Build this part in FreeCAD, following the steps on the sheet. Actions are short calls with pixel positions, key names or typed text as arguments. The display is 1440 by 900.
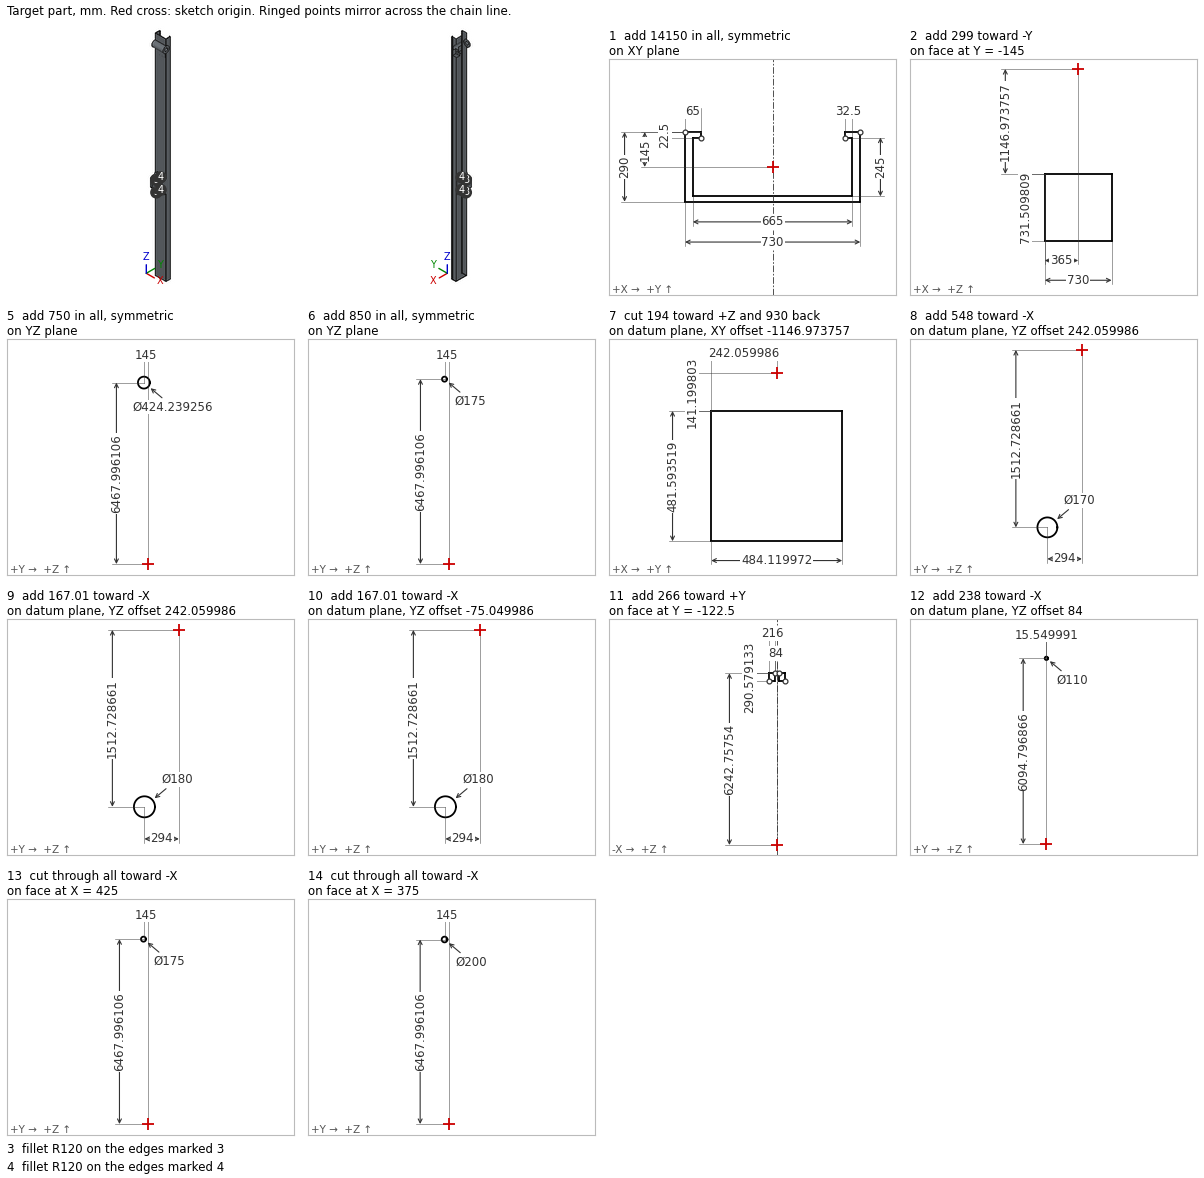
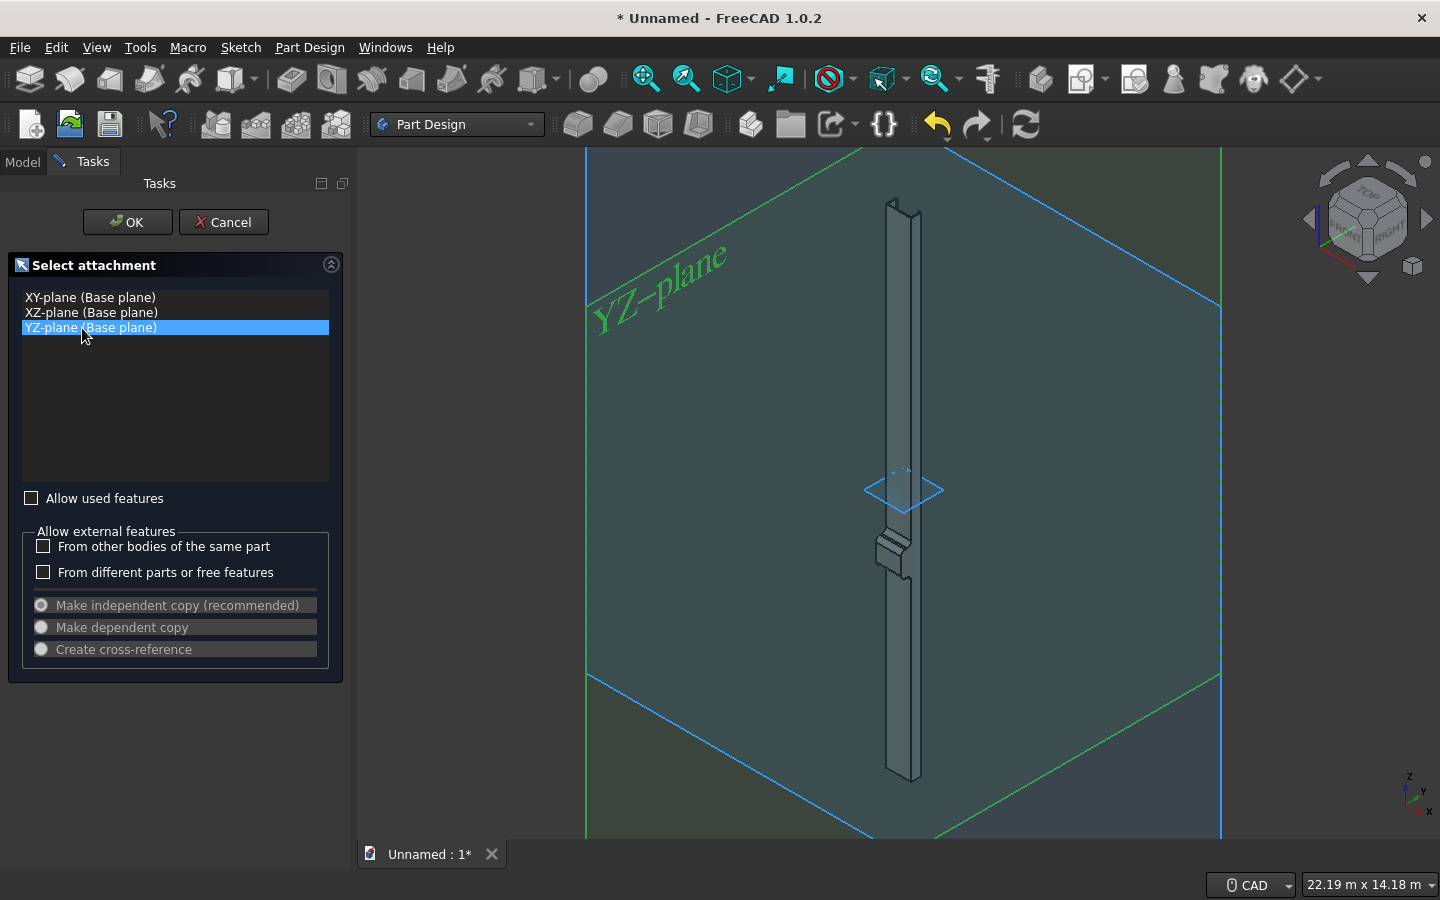
click(128, 222)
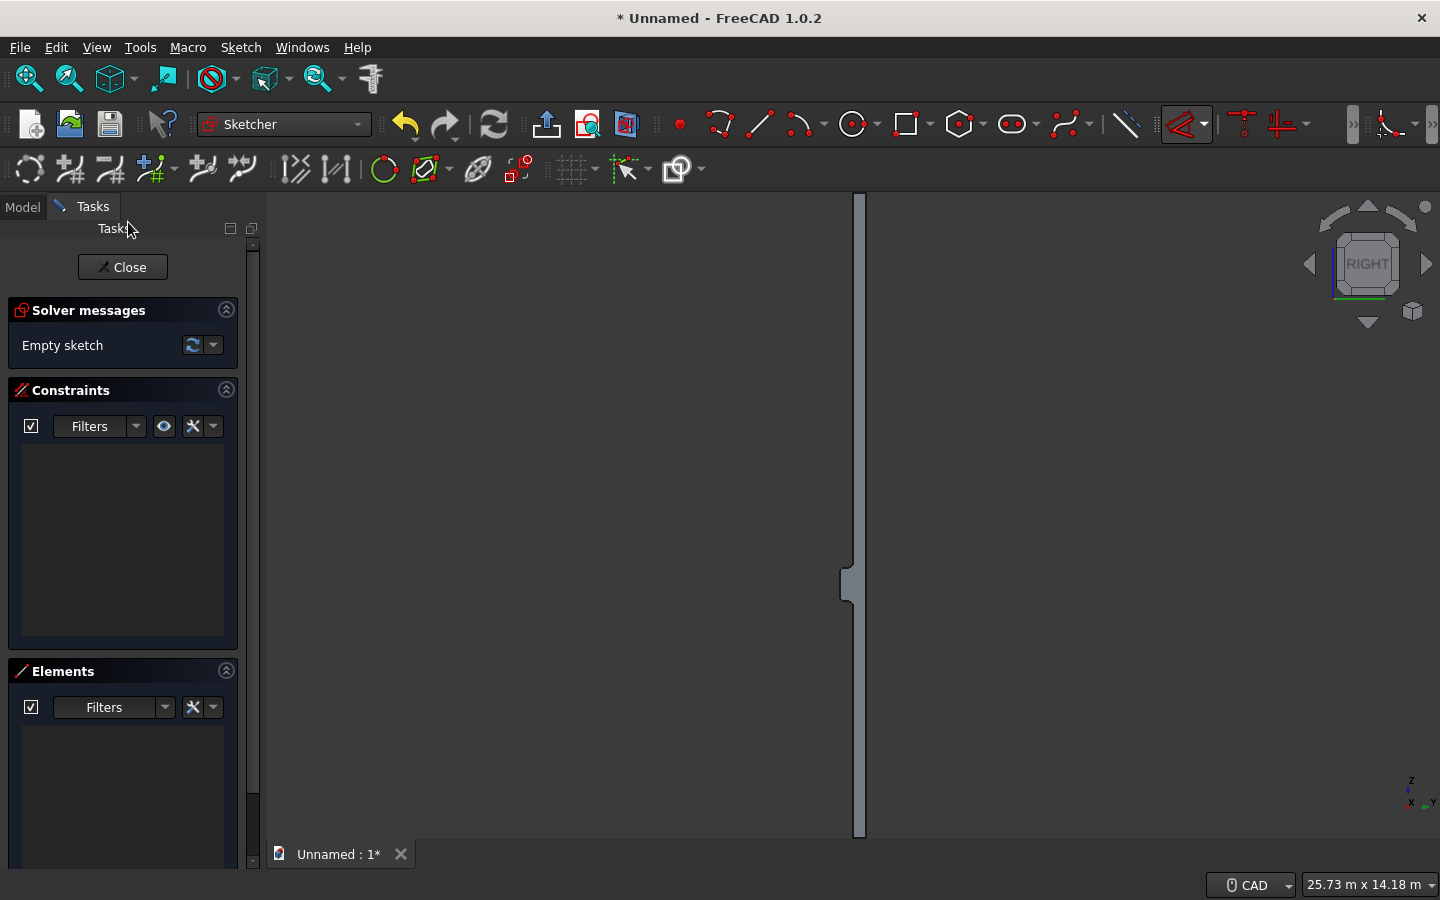
key(q)
key(s)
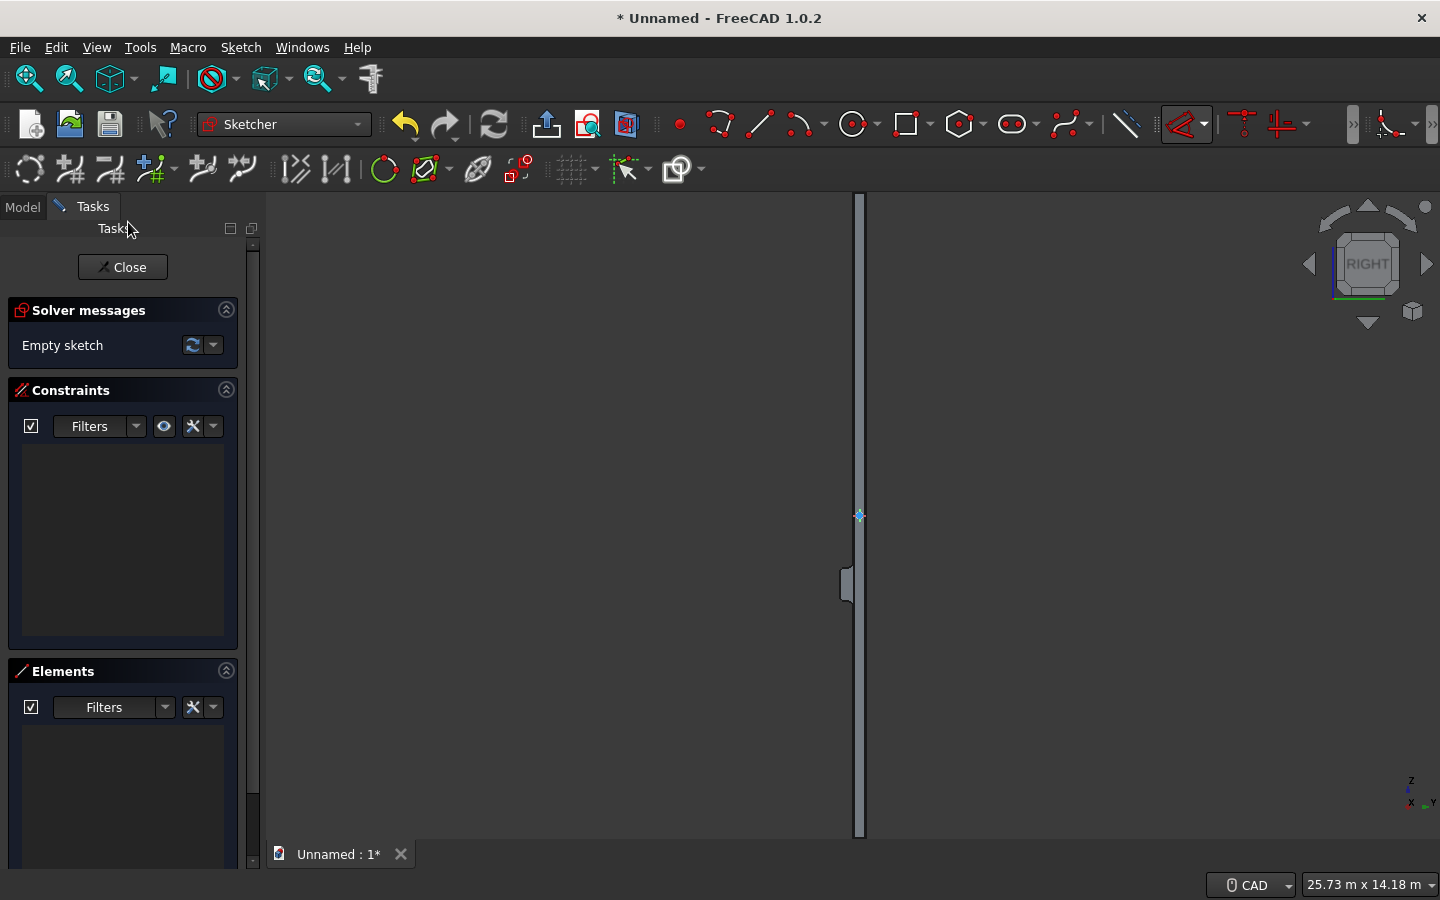
scroll(784, 516, down, 5)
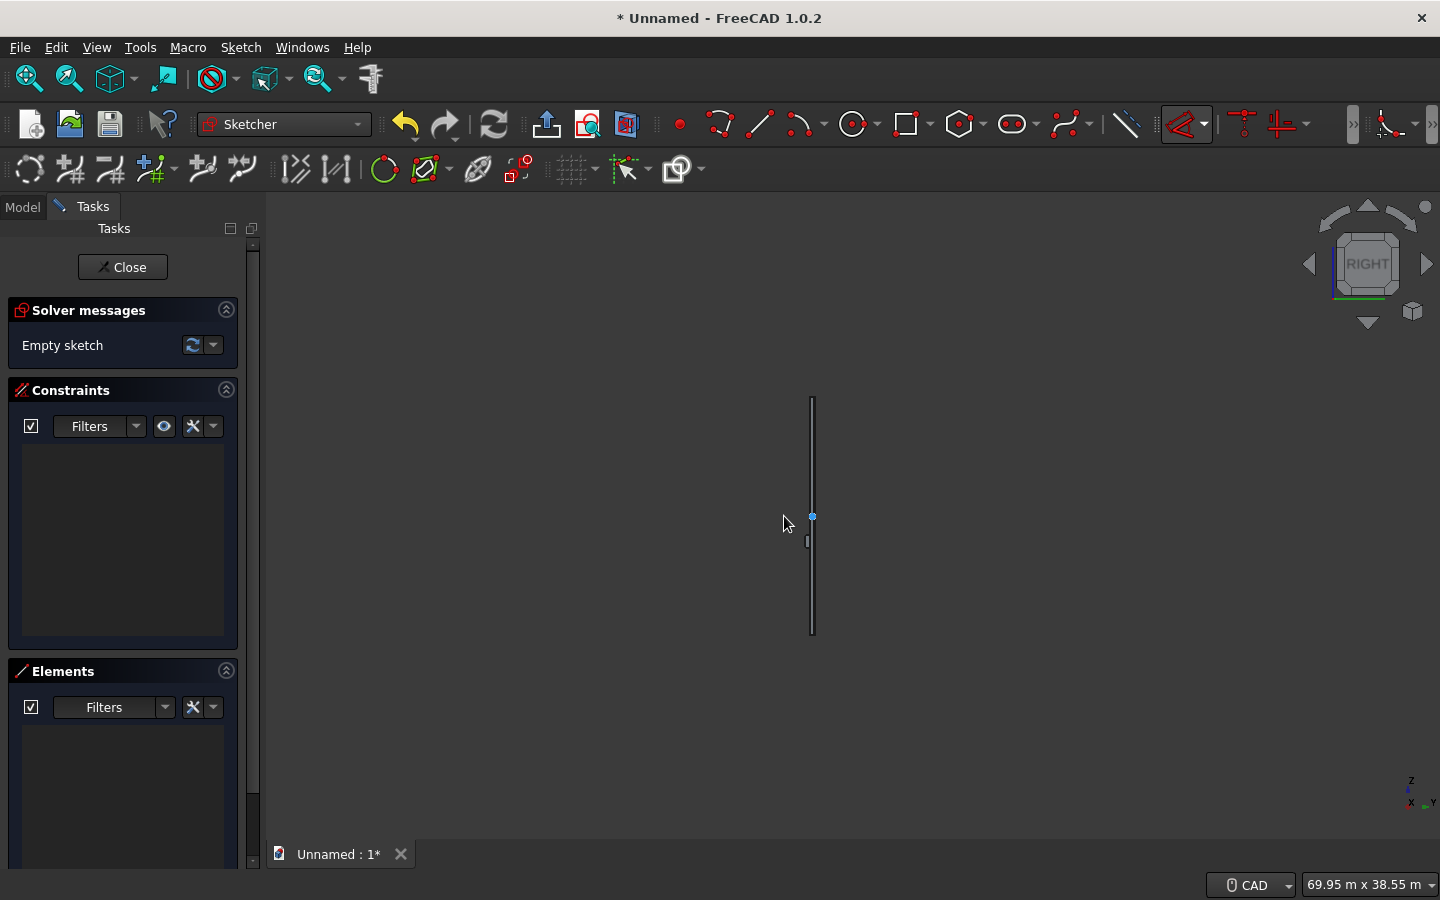
scroll(811, 402, up, 15)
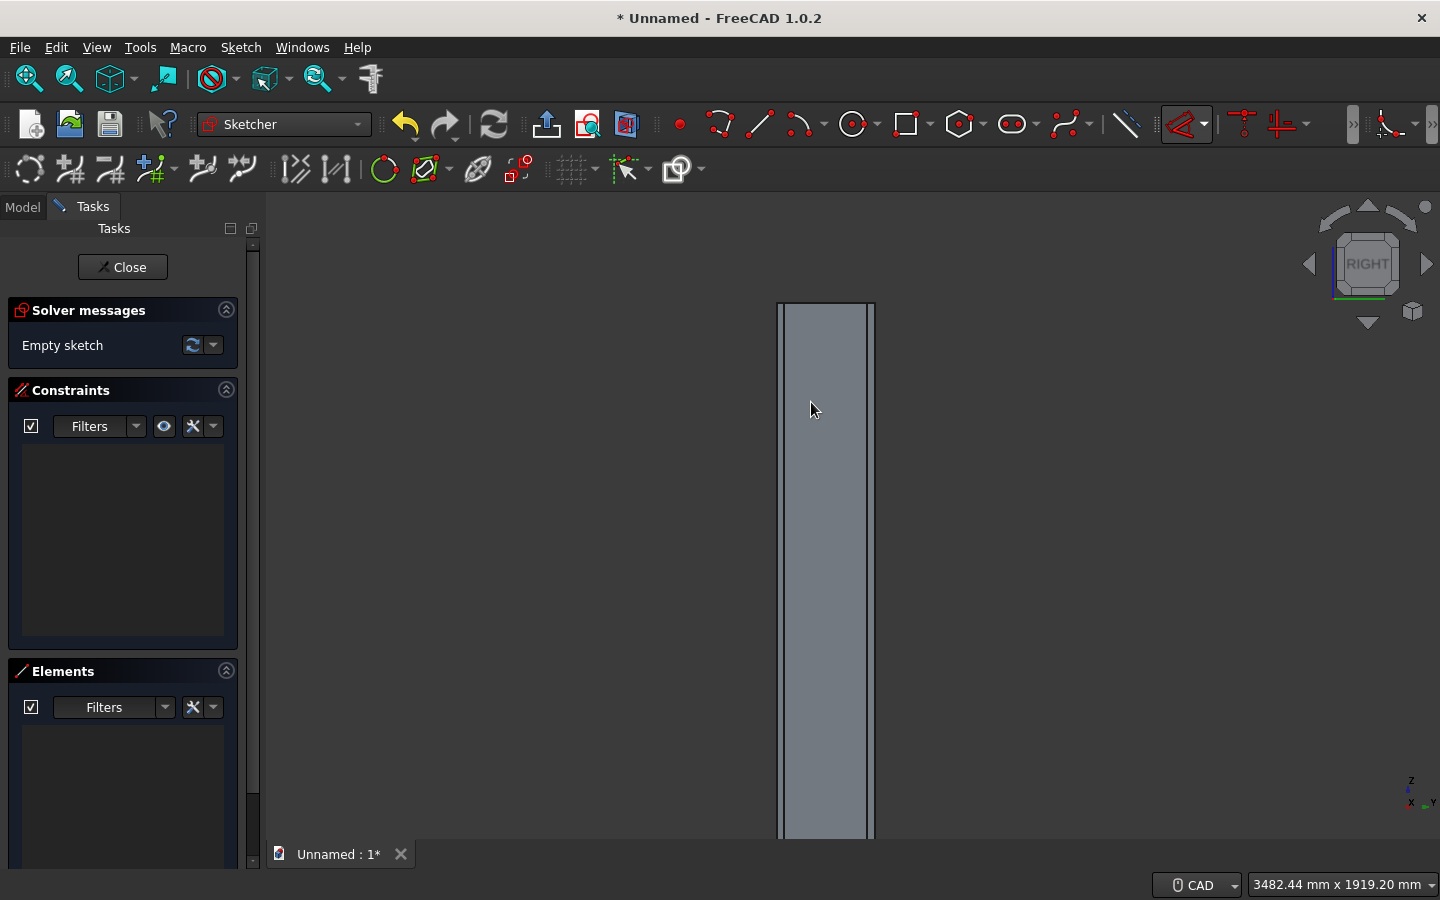
scroll(772, 503, up, 5)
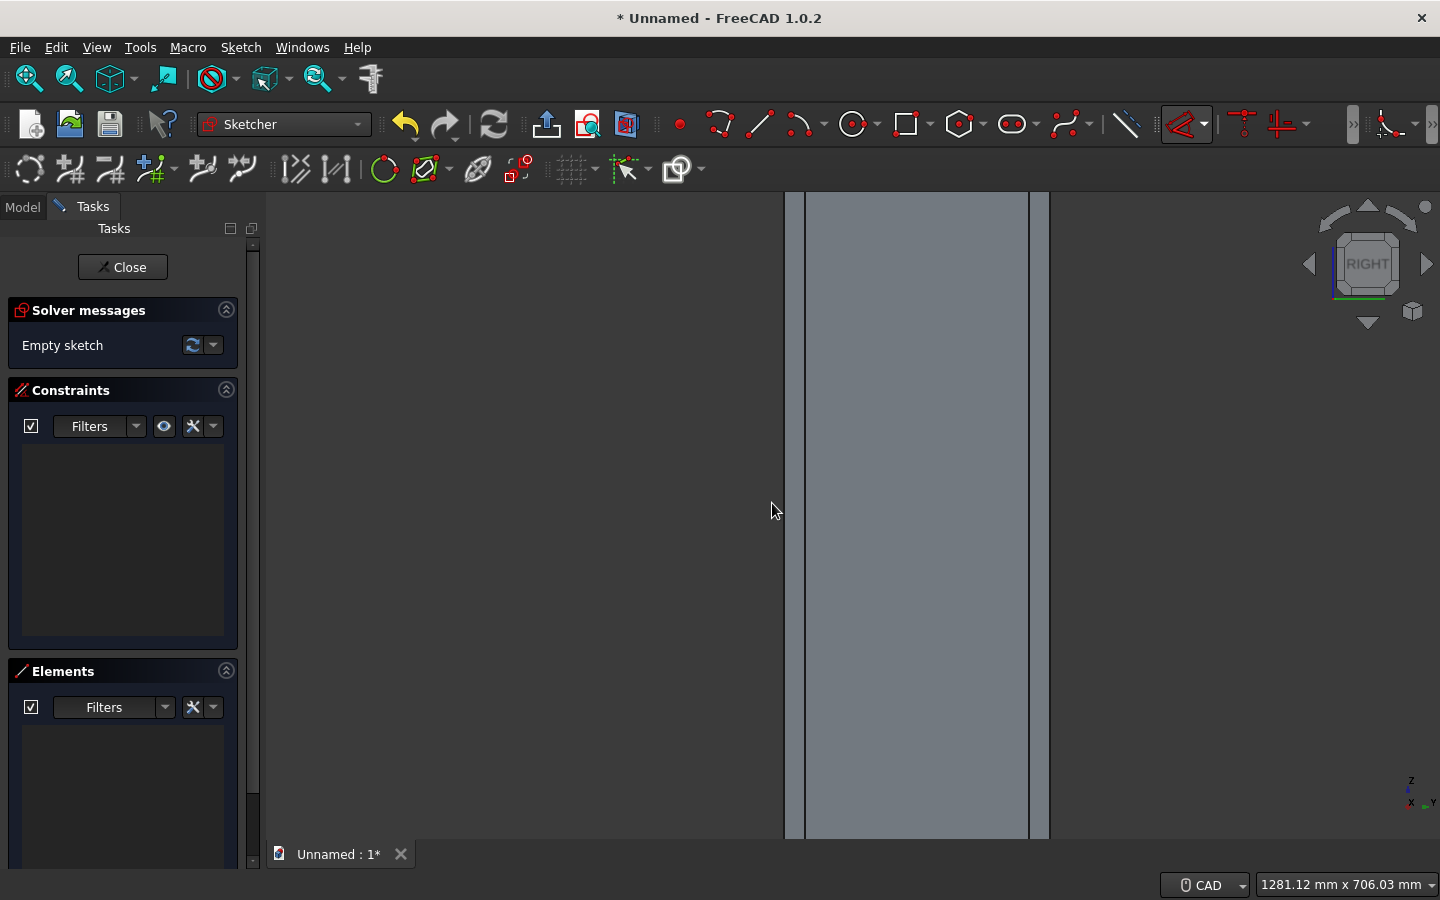
key(g)
key(c)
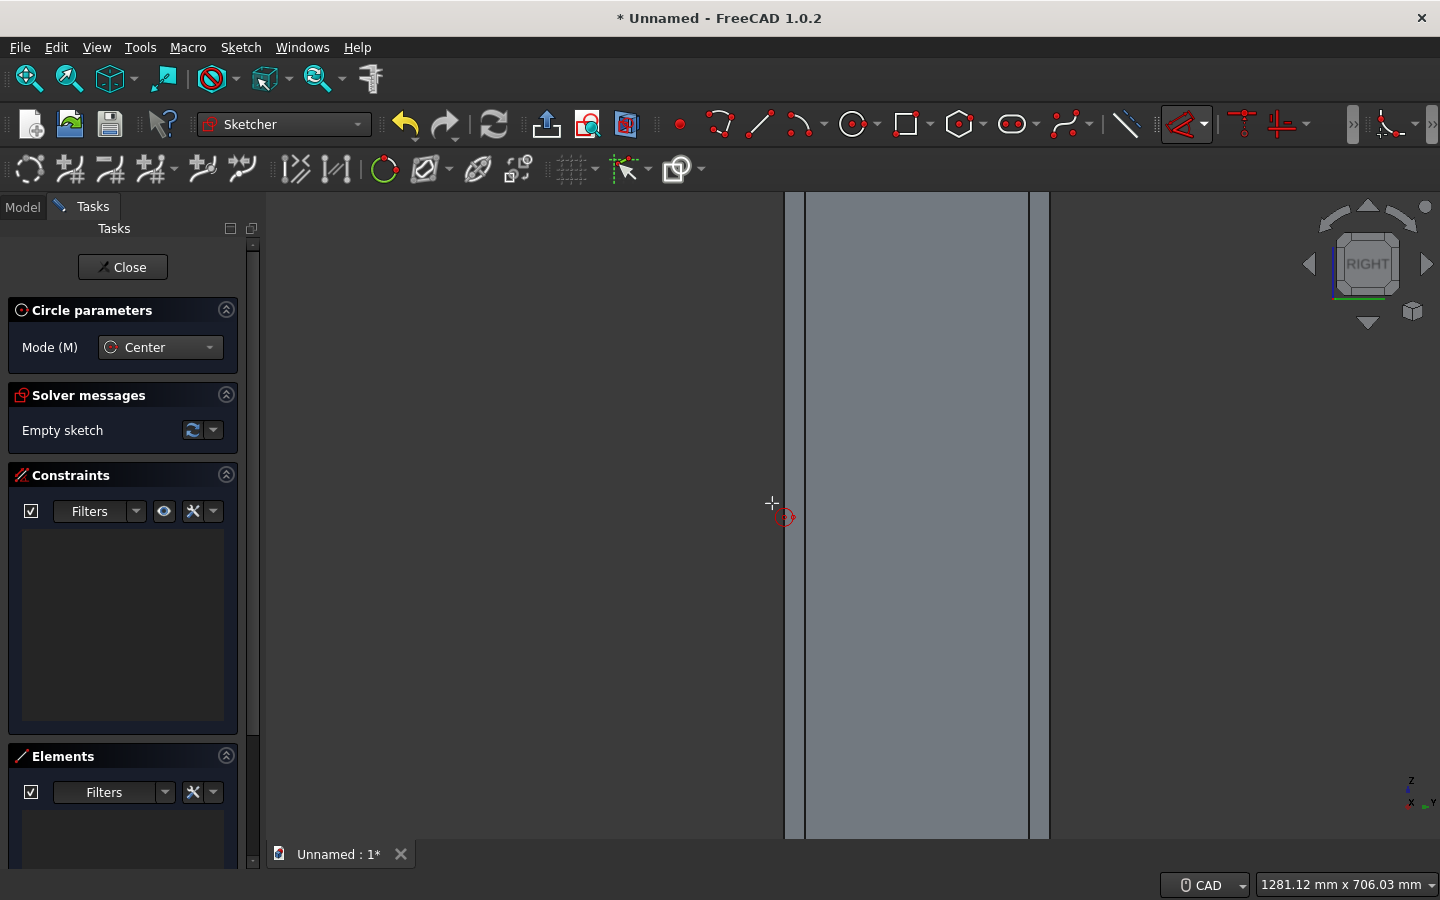
click(784, 515)
click(647, 378)
key(Escape)